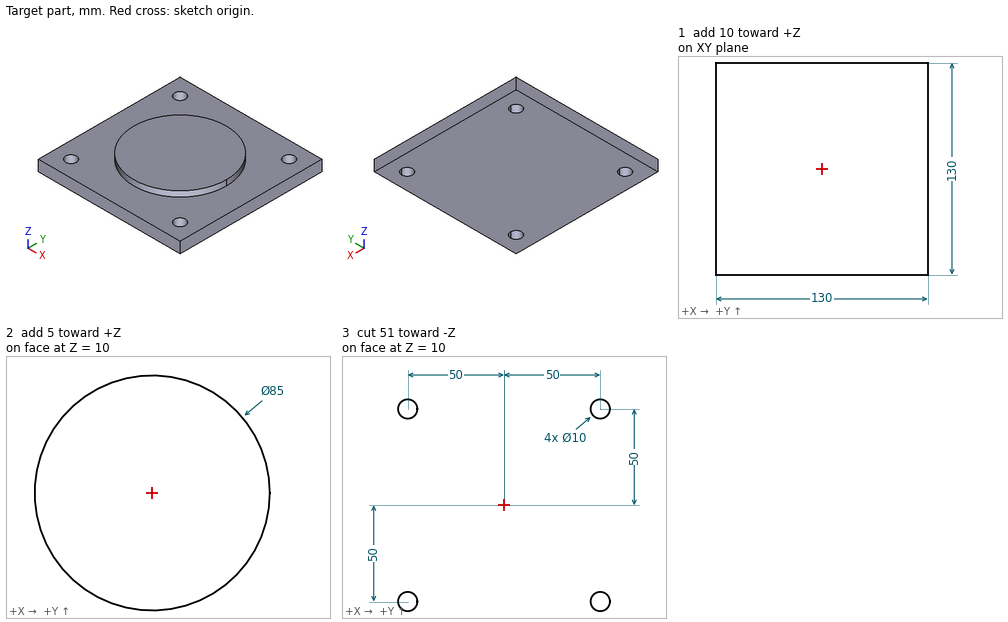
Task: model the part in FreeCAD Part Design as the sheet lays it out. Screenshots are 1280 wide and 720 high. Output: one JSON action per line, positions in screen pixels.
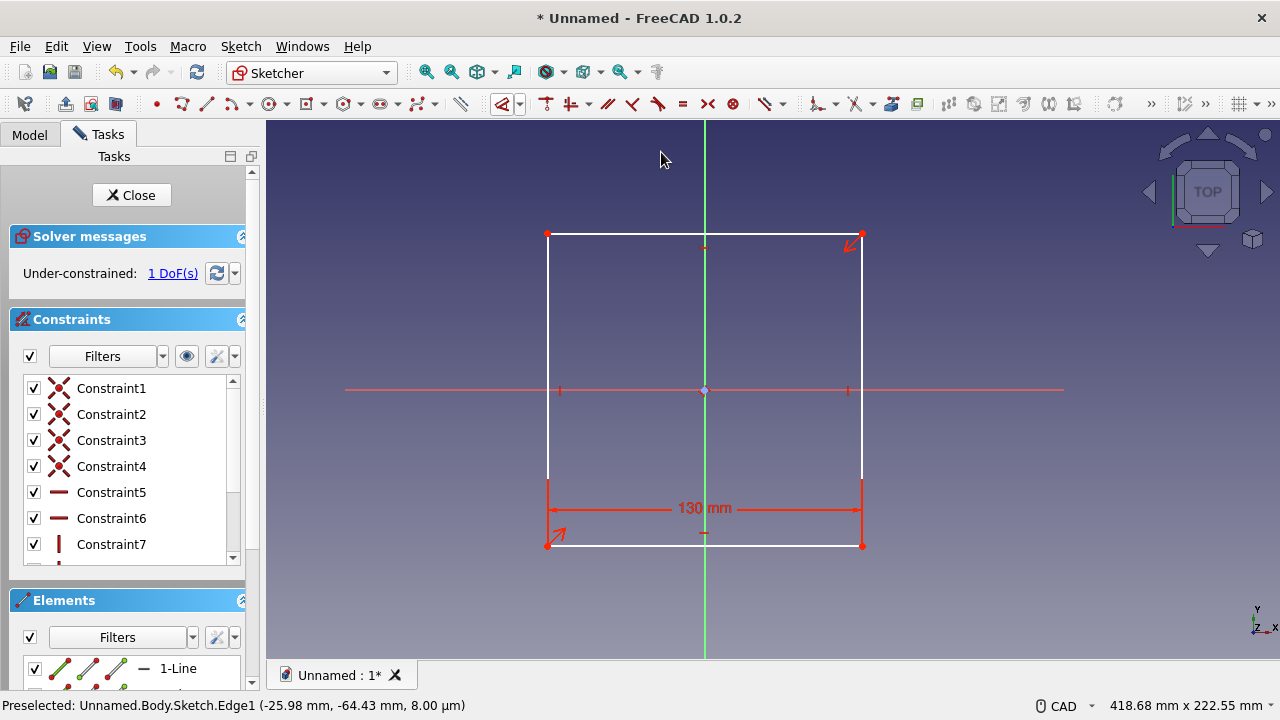
{"action": "left_click", "coordinate": [862, 452]}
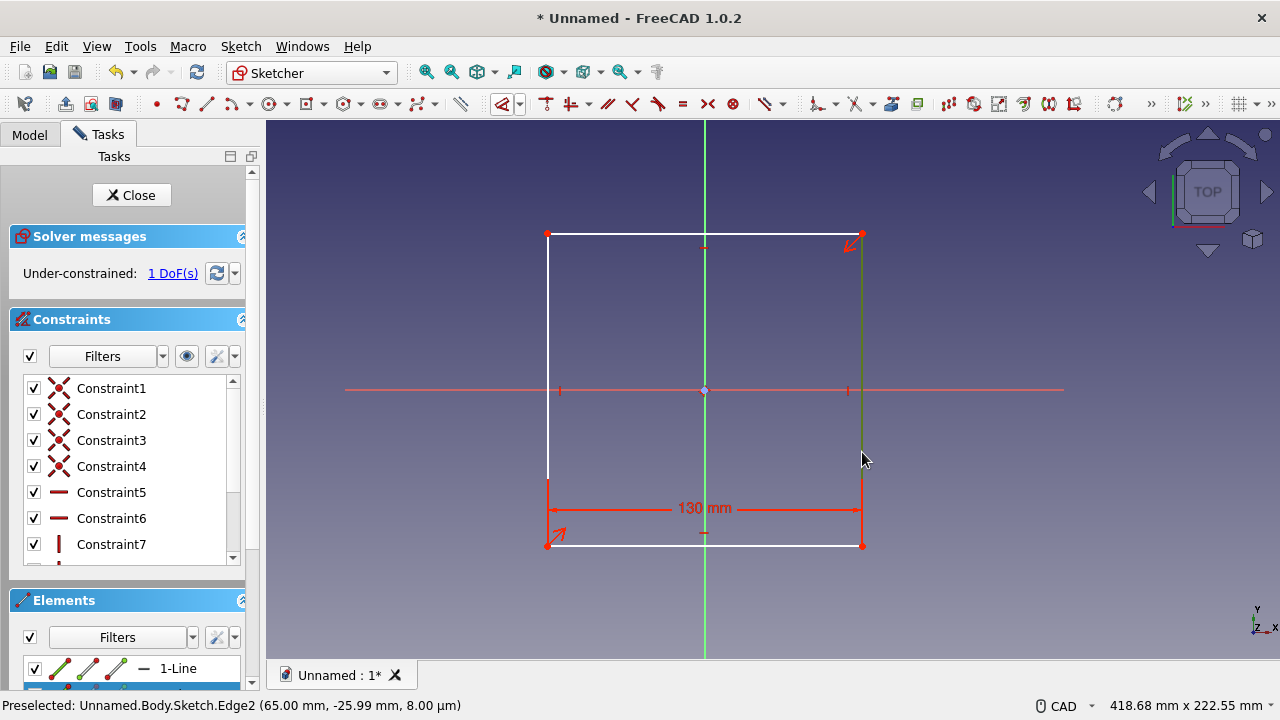
{"action": "left_click", "coordinate": [520, 104]}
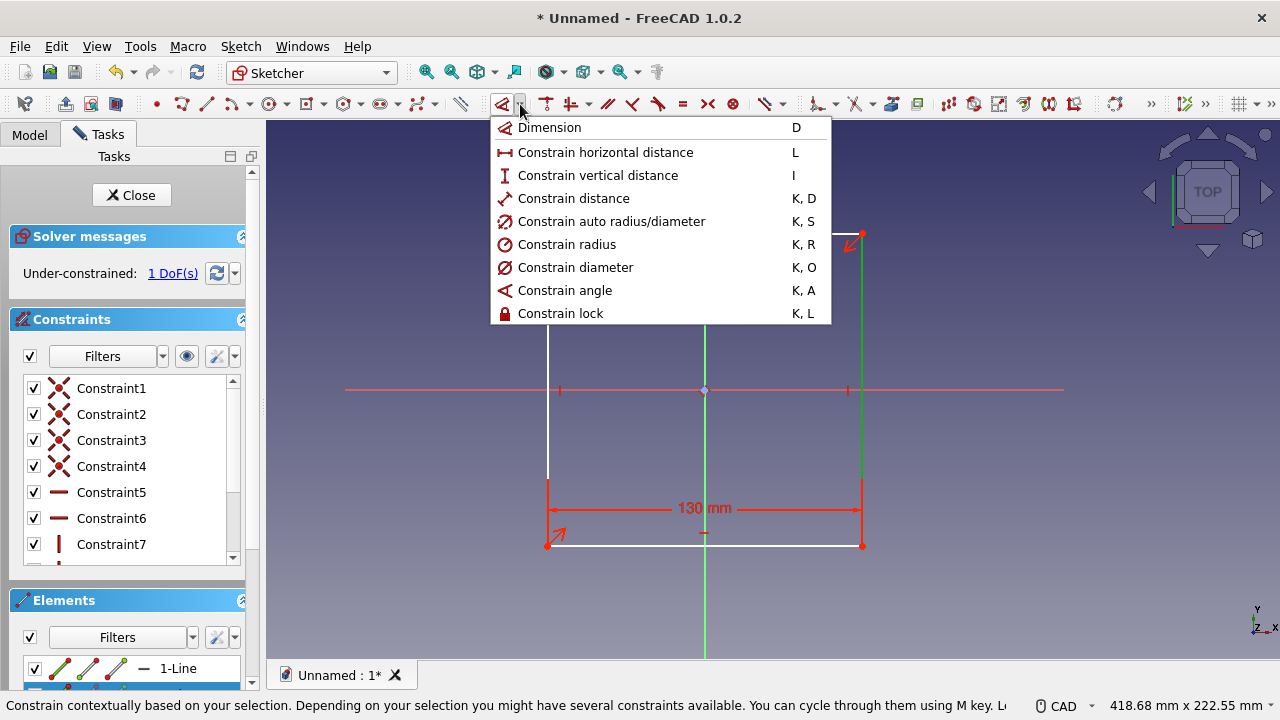
{"action": "left_click", "coordinate": [661, 176]}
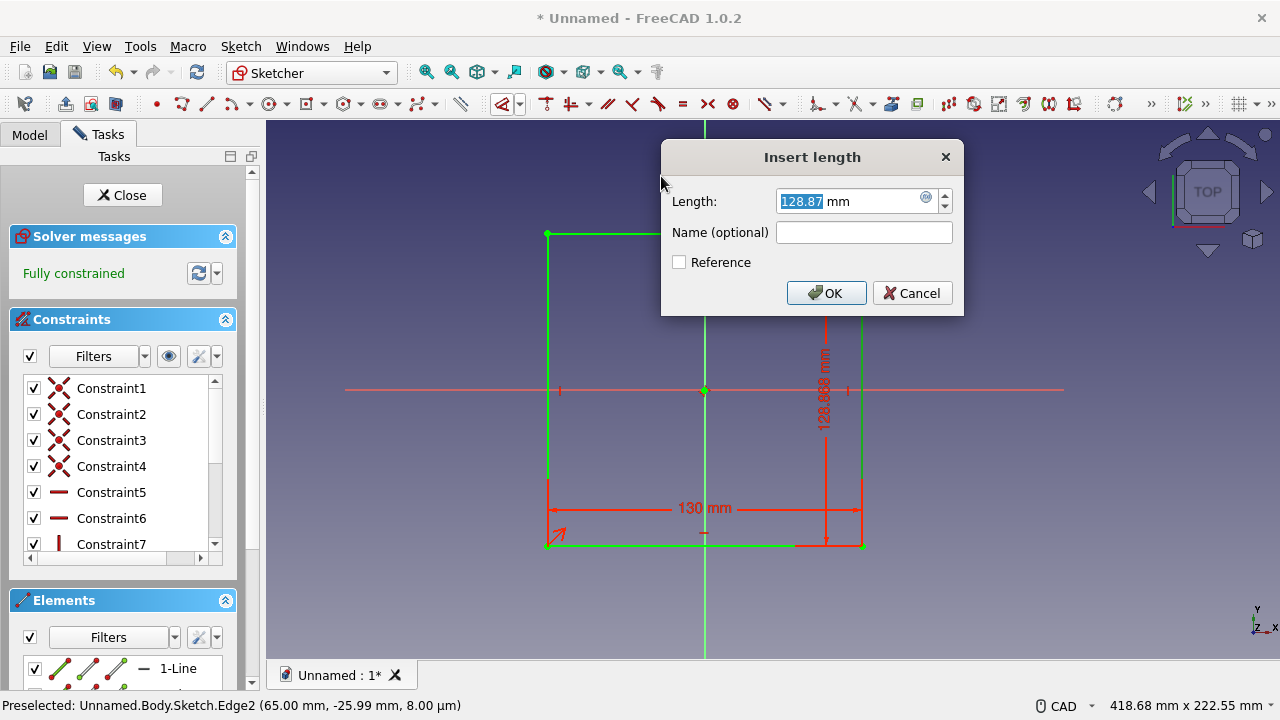
{"action": "type", "text": "130"}
{"action": "key", "text": "Return"}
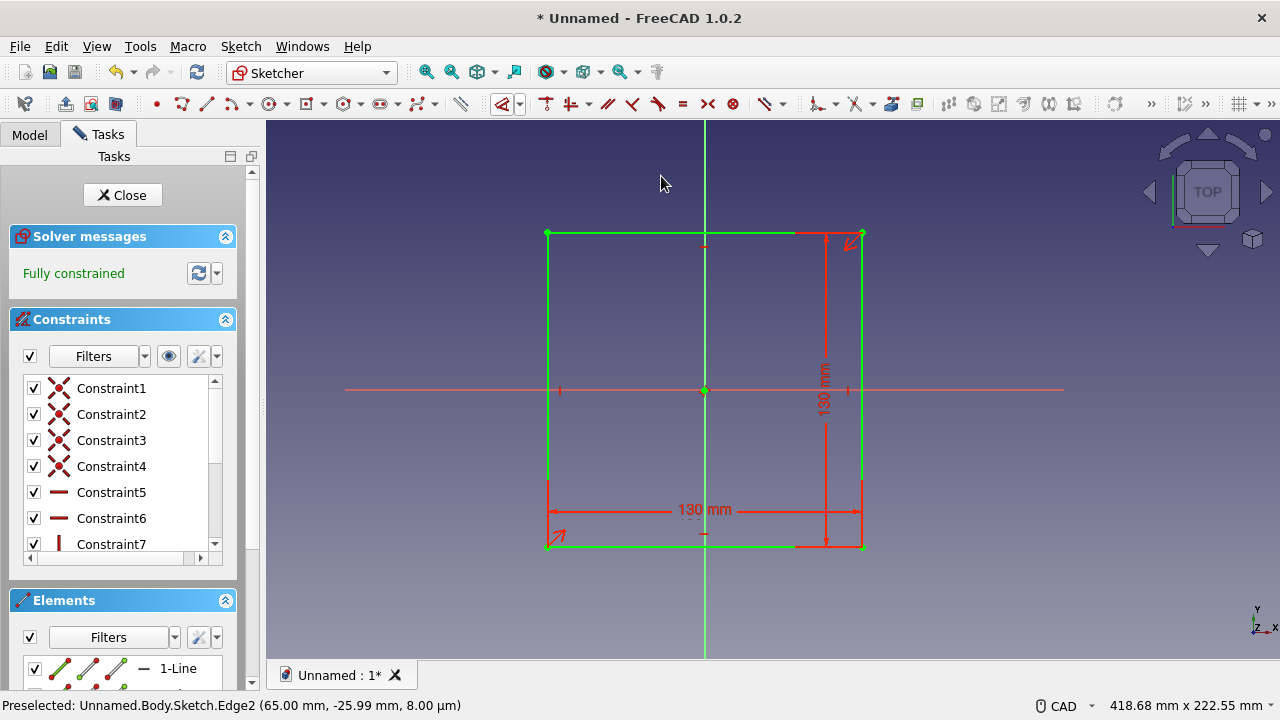
{"action": "left_click", "coordinate": [123, 195]}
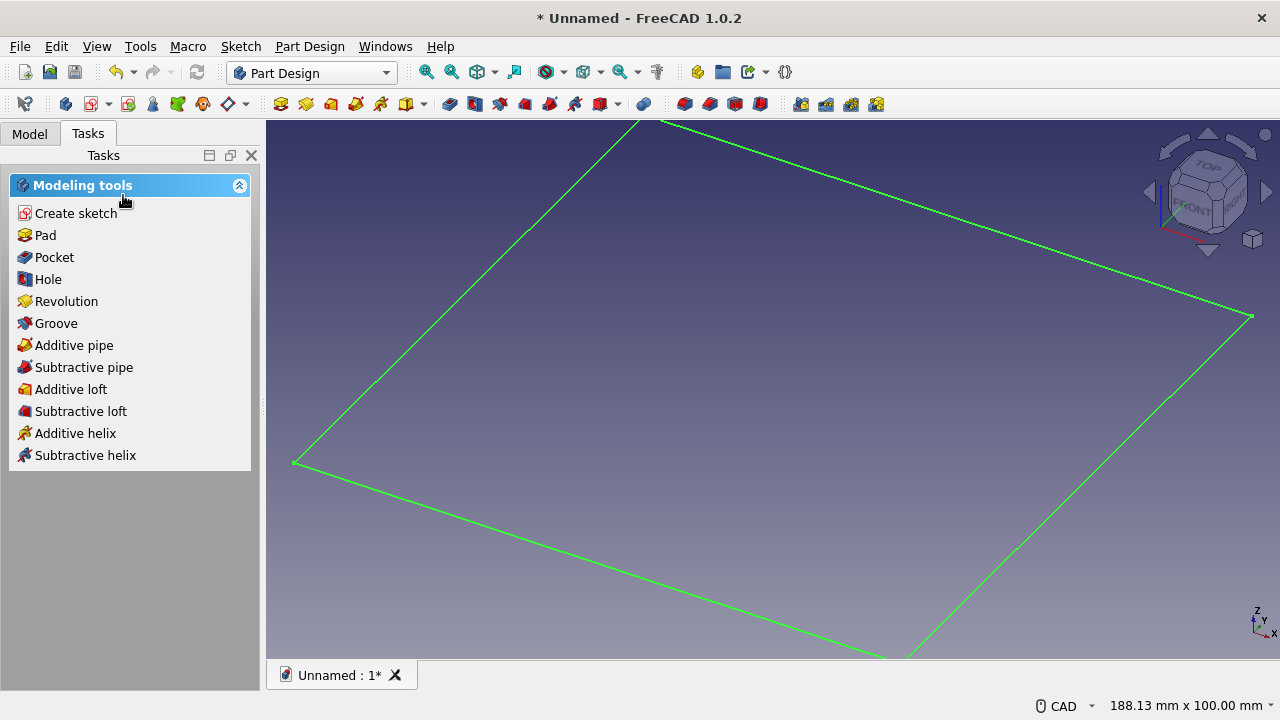
{"action": "left_click", "coordinate": [281, 104]}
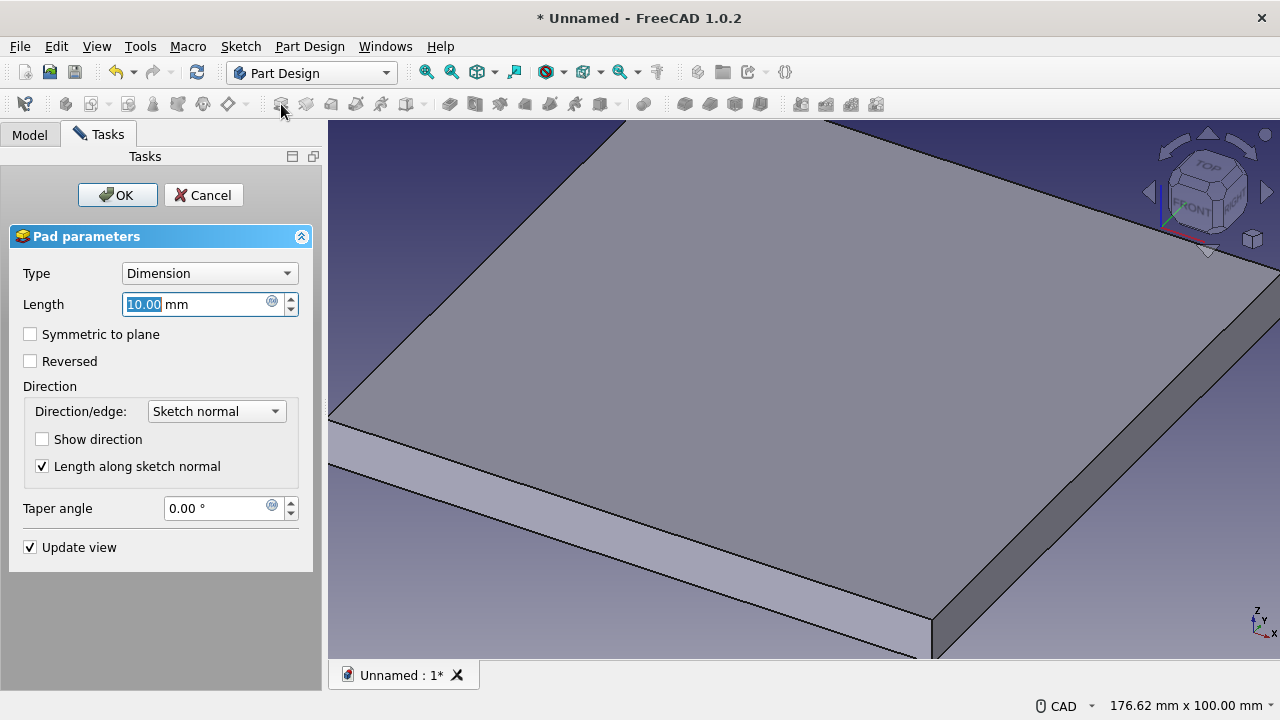
{"action": "type", "text": "10"}
{"action": "key", "text": "Tab"}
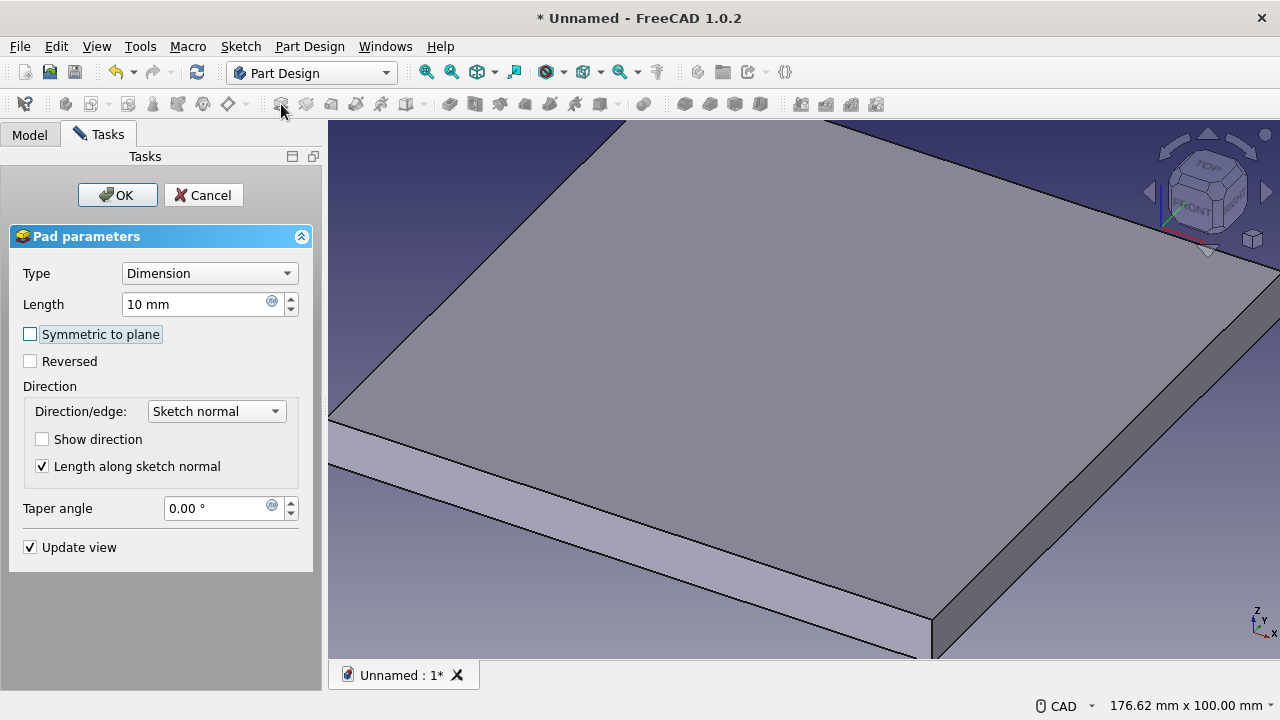
{"action": "left_click", "coordinate": [118, 195]}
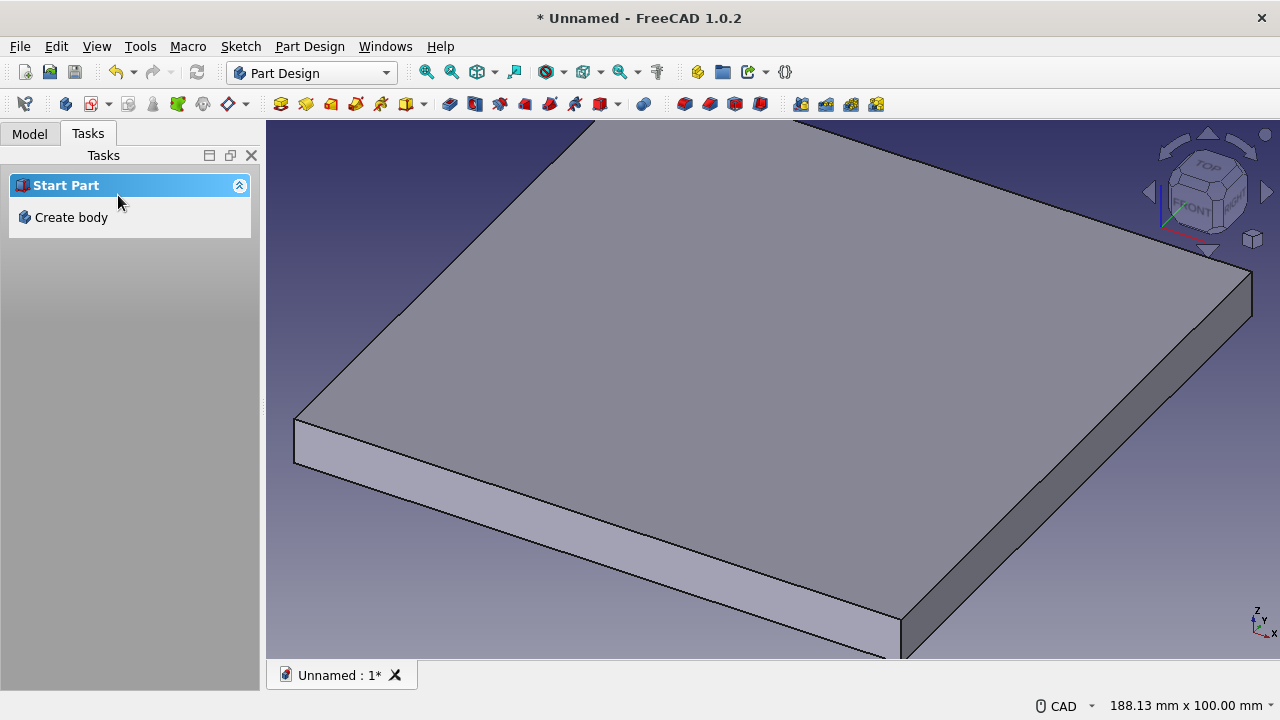
{"action": "left_click", "coordinate": [427, 72]}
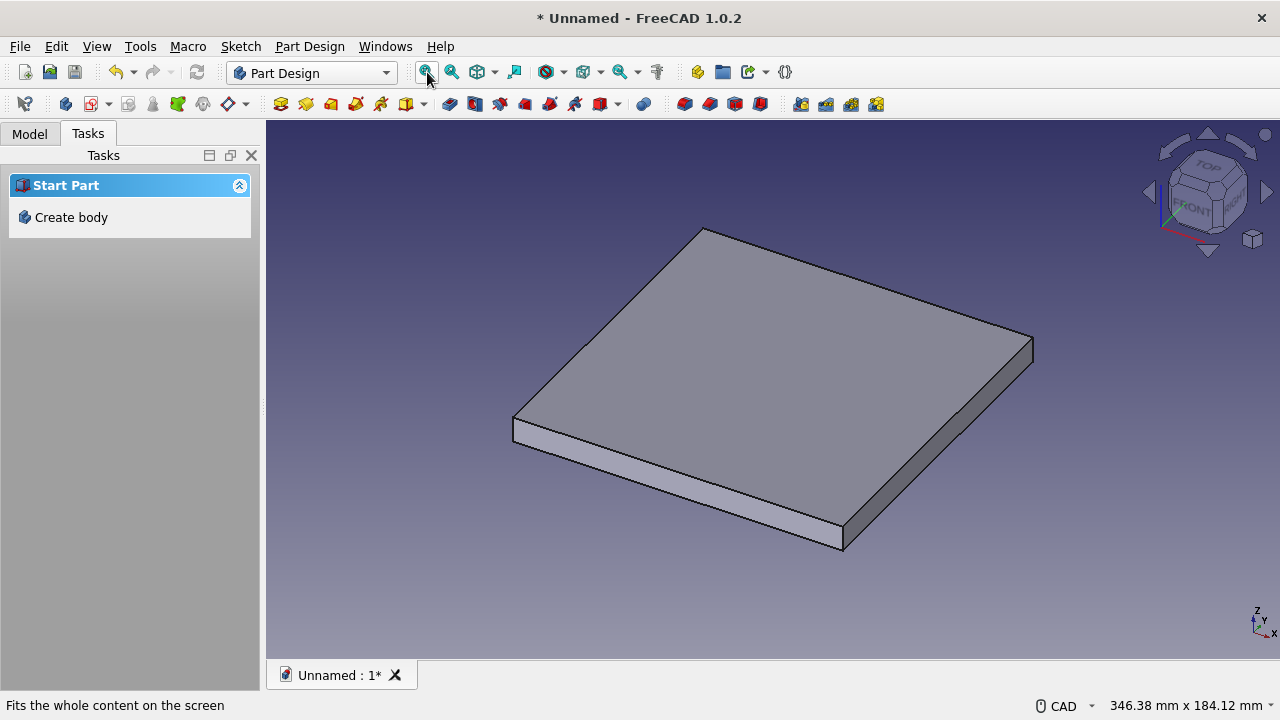
{"action": "left_click", "coordinate": [773, 377]}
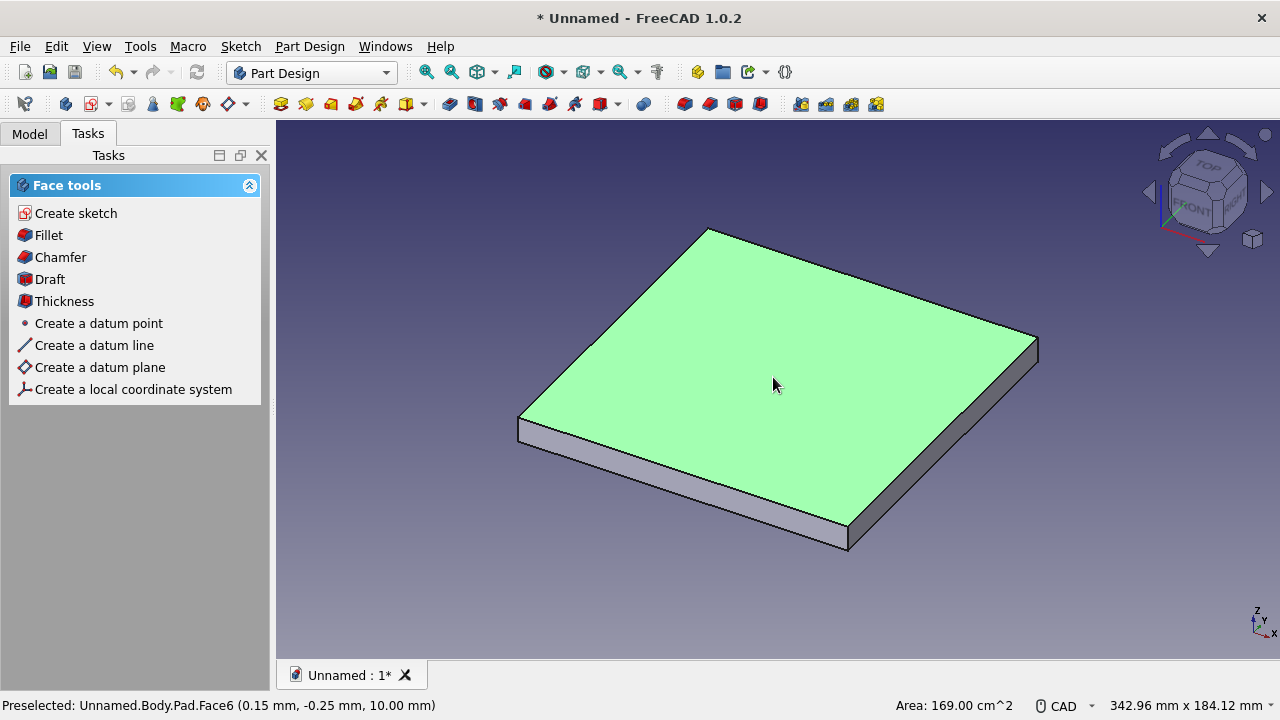
{"action": "left_click", "coordinate": [90, 104]}